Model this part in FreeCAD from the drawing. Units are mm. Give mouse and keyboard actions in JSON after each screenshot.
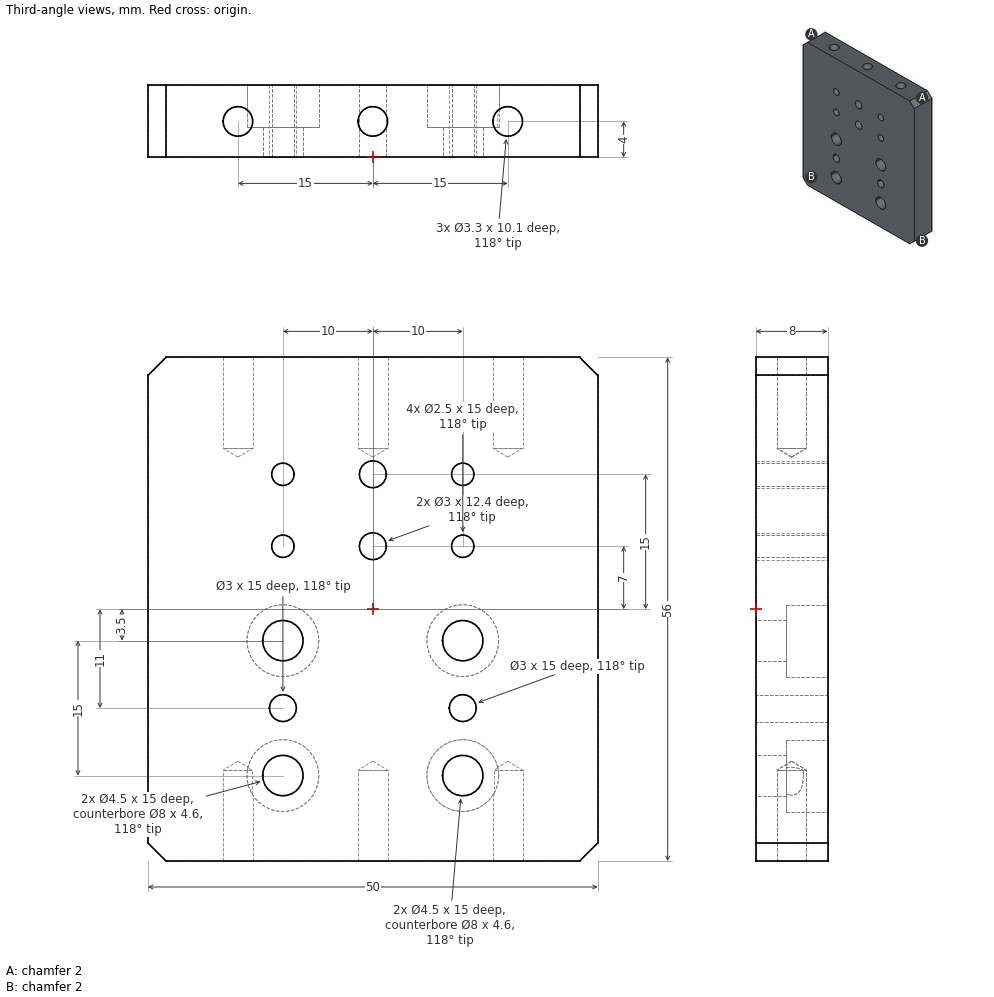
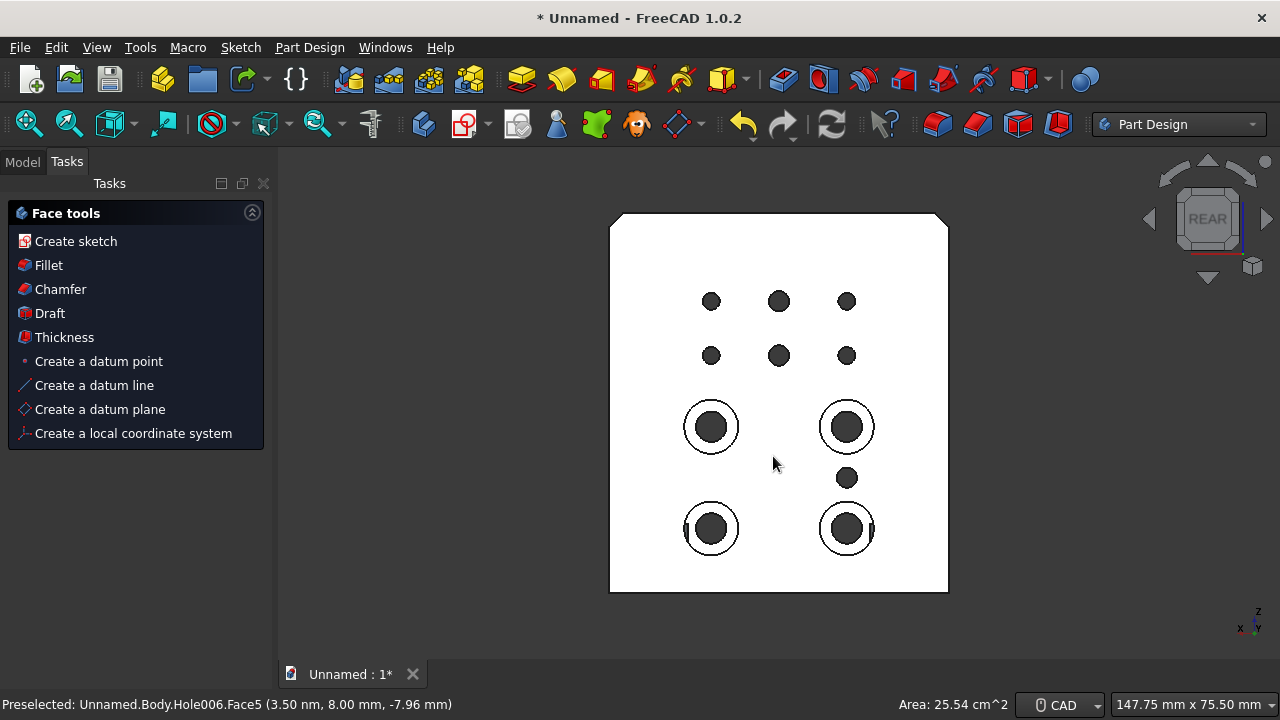
{"action": "left_click", "coordinate": [464, 124]}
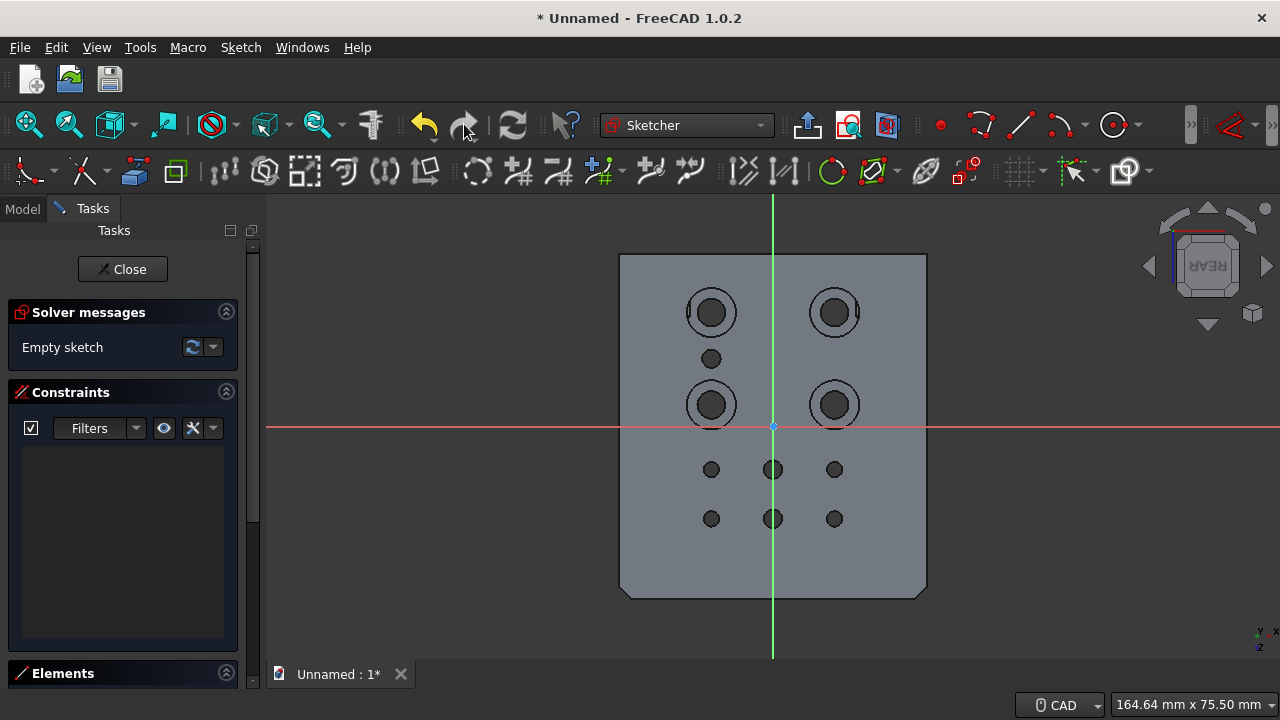
{"action": "scroll", "coordinate": [843, 354], "scroll_direction": "up", "scroll_amount": 14}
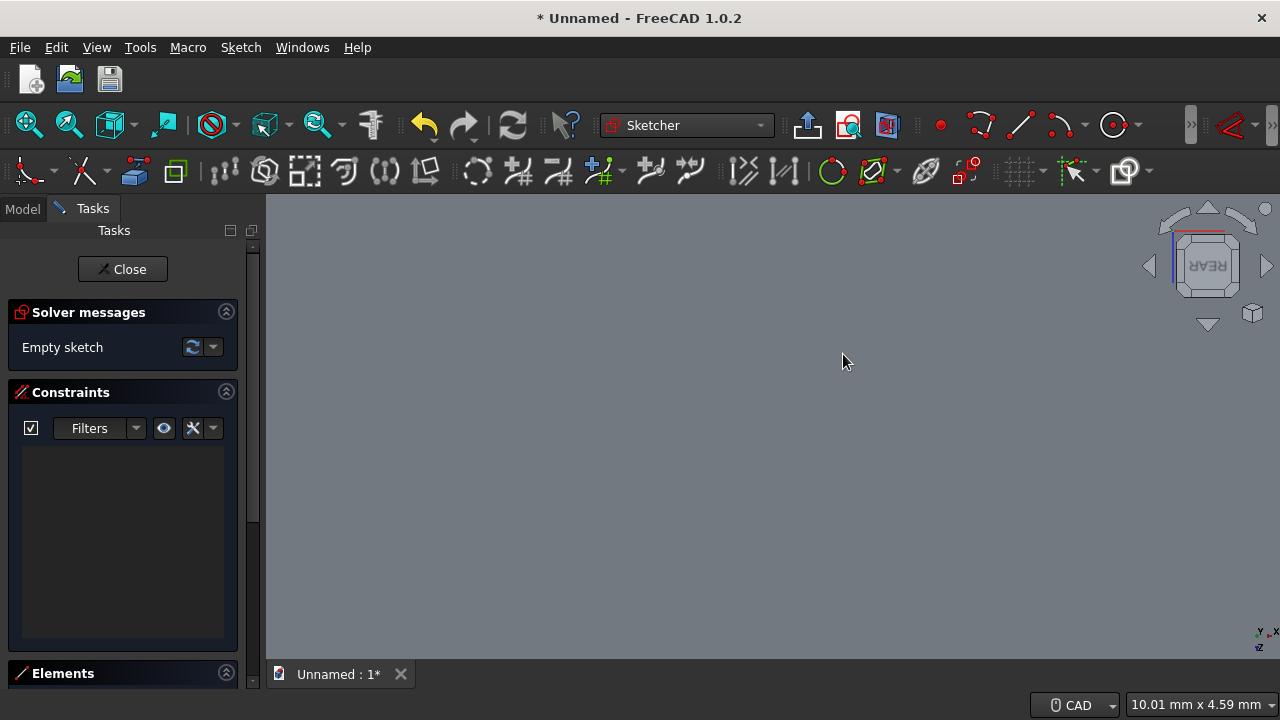
{"action": "left_click", "coordinate": [1114, 126]}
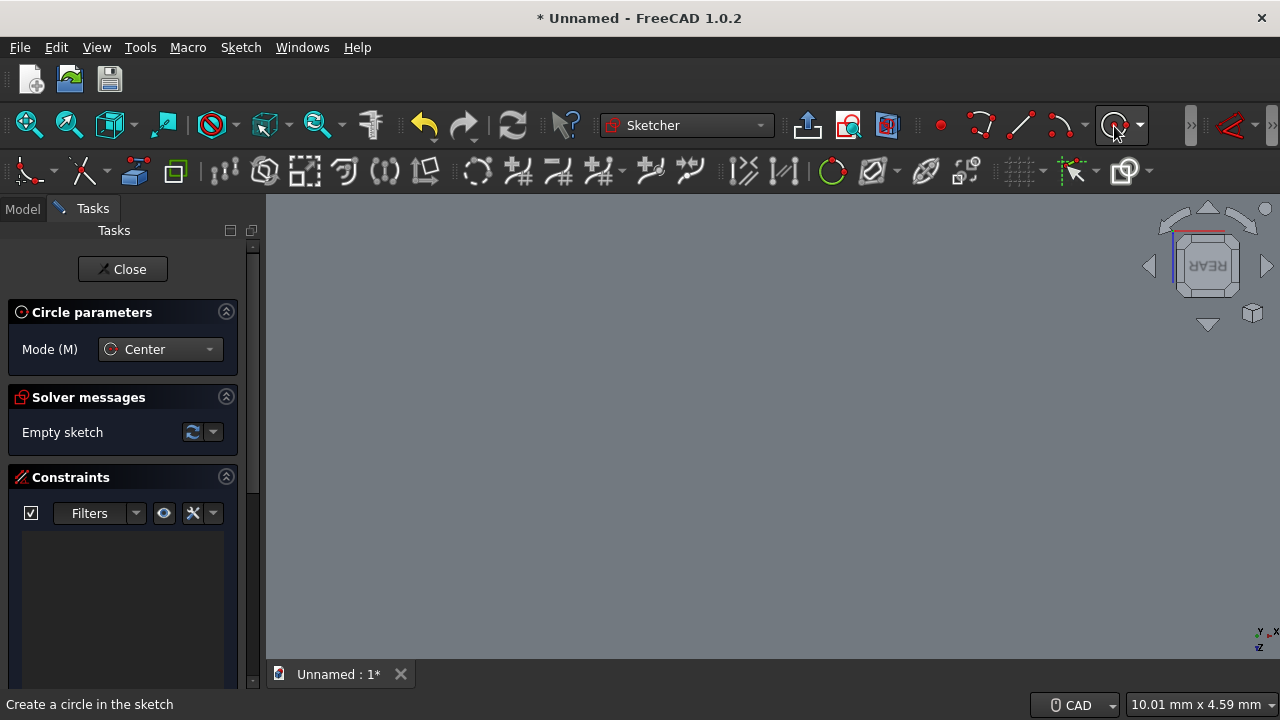
{"action": "left_click", "coordinate": [696, 427]}
{"action": "mouse_move", "coordinate": [803, 319]}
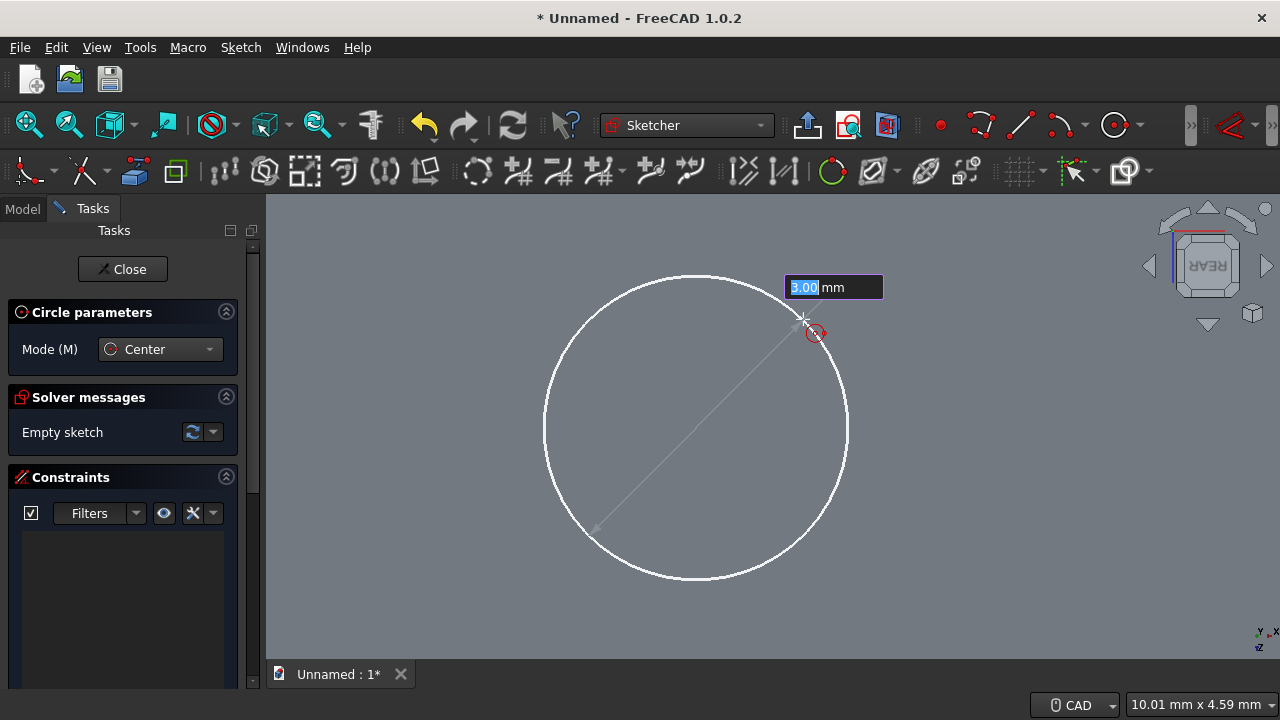
{"action": "type", "text": "3"}
{"action": "key", "text": "Return"}
{"action": "key", "text": "Escape"}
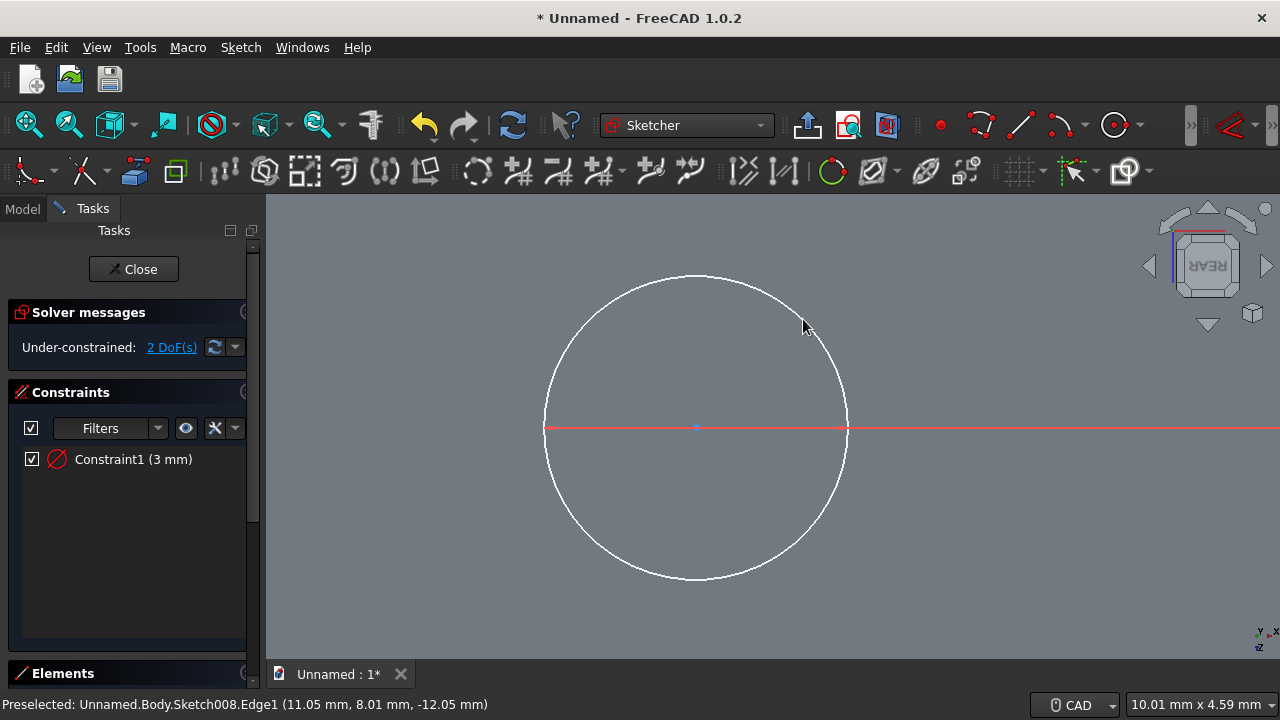
{"action": "key", "text": "d"}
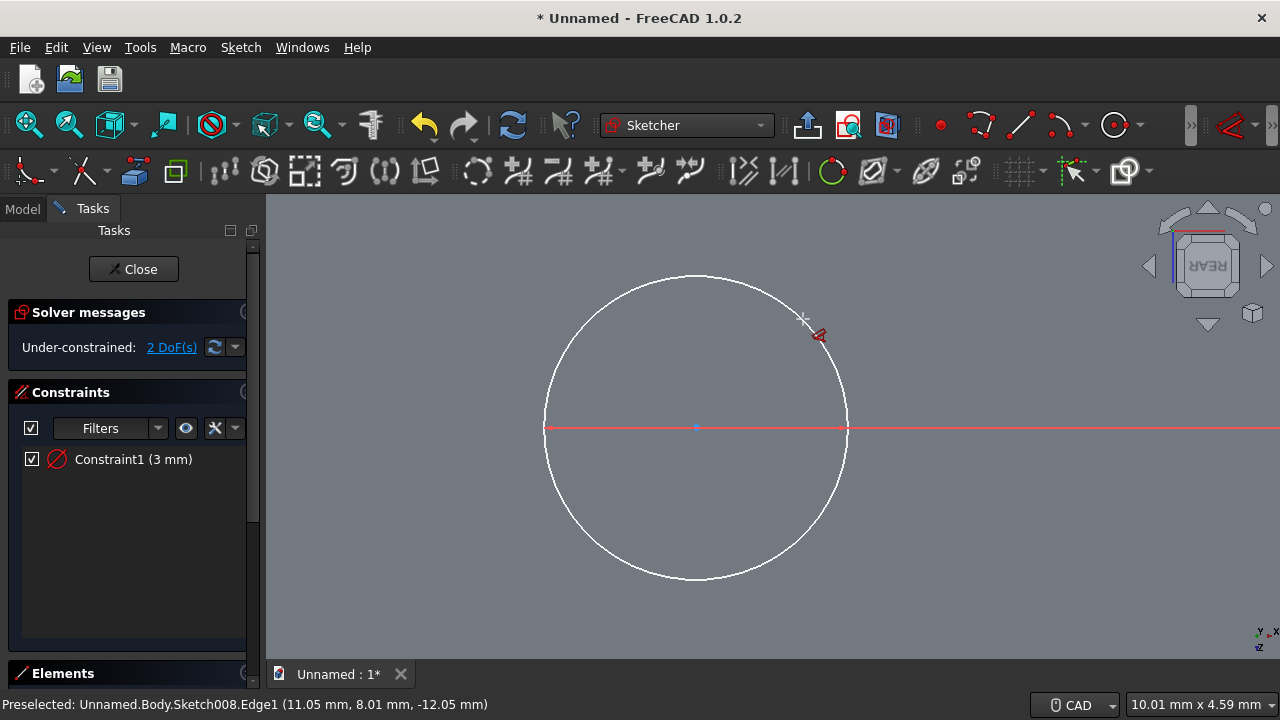
{"action": "left_click", "coordinate": [696, 428]}
{"action": "left_click", "coordinate": [495, 394]}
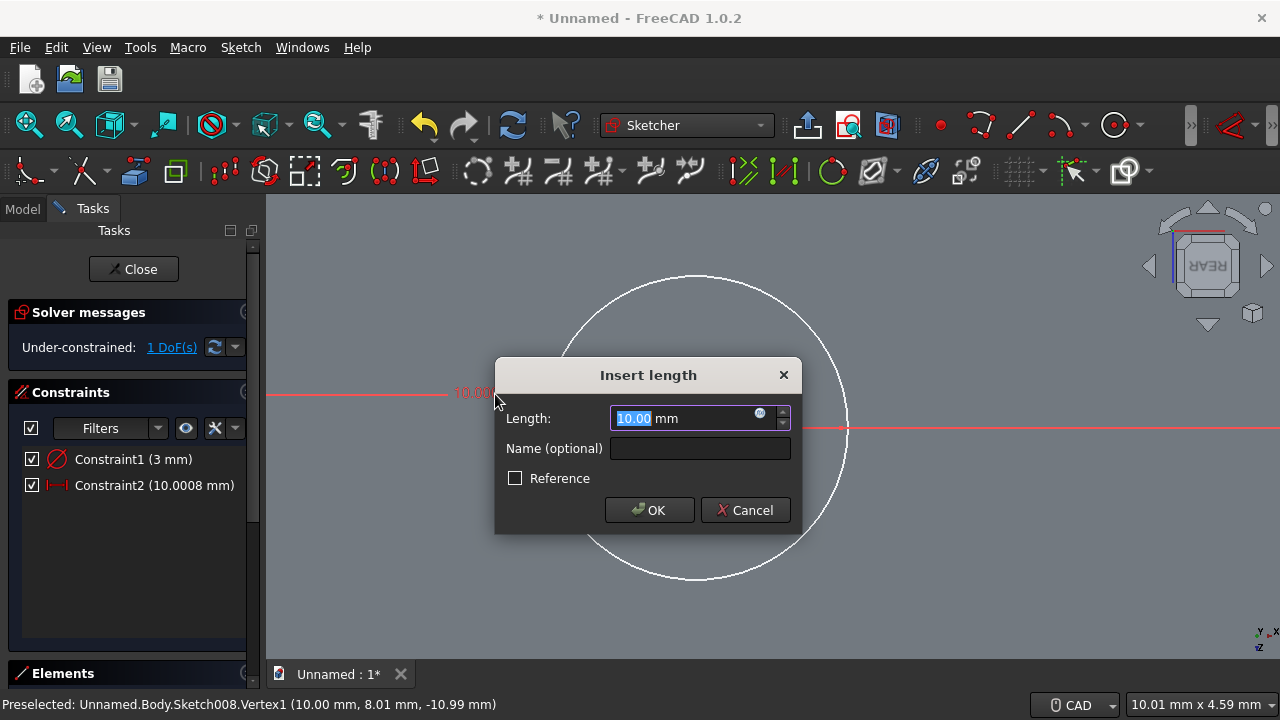
{"action": "type", "text": "10"}
{"action": "key", "text": "Return"}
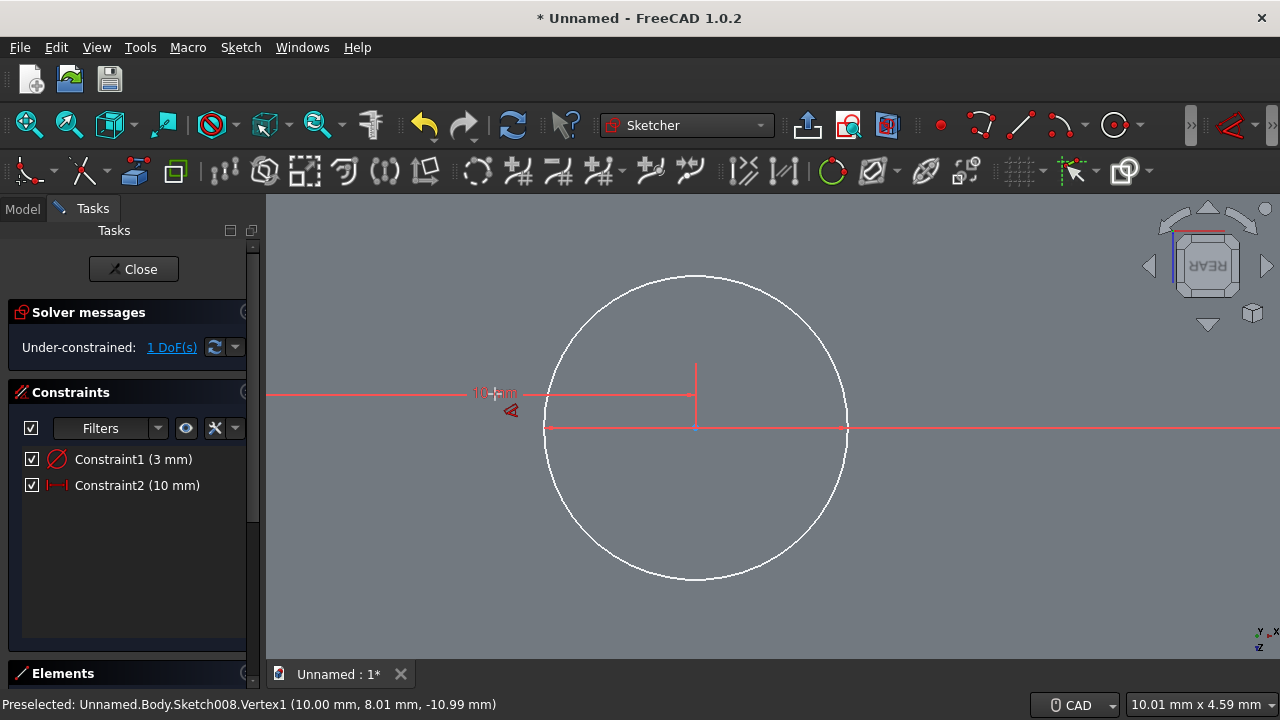
{"action": "left_click", "coordinate": [696, 428]}
{"action": "left_click", "coordinate": [730, 529]}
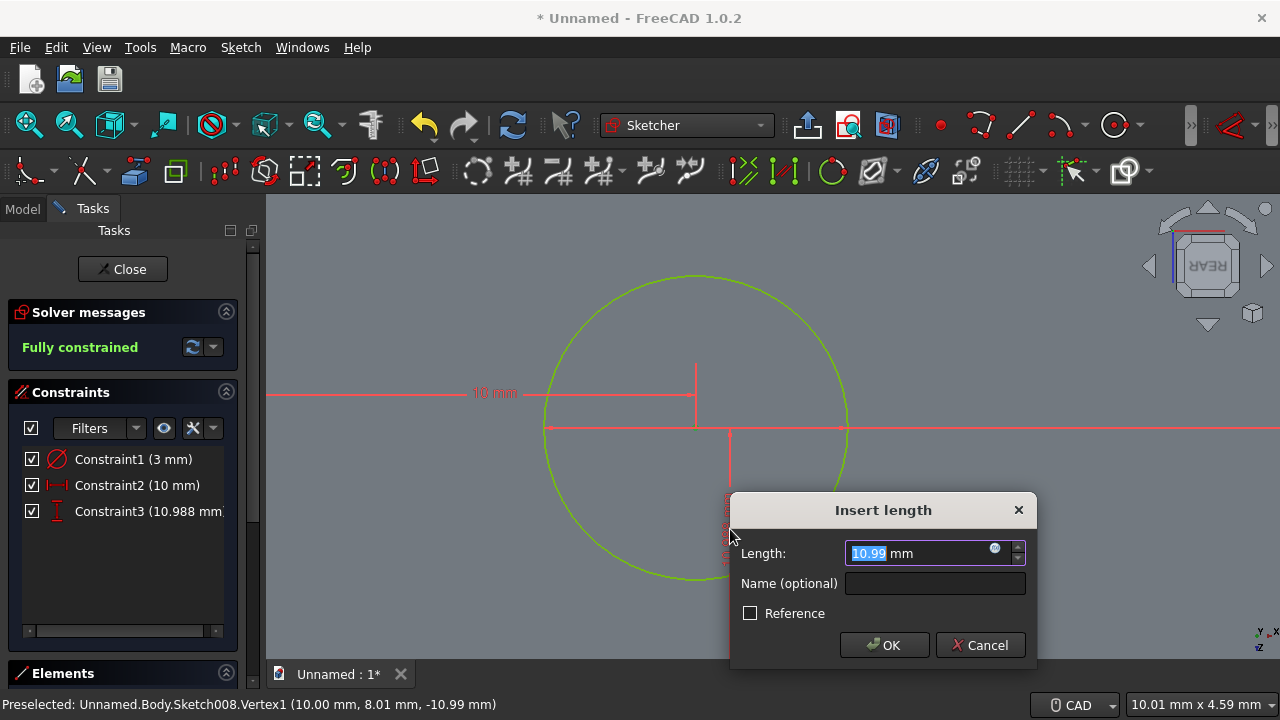
{"action": "type", "text": "11"}
{"action": "key", "text": "Return"}
{"action": "key", "text": "Escape"}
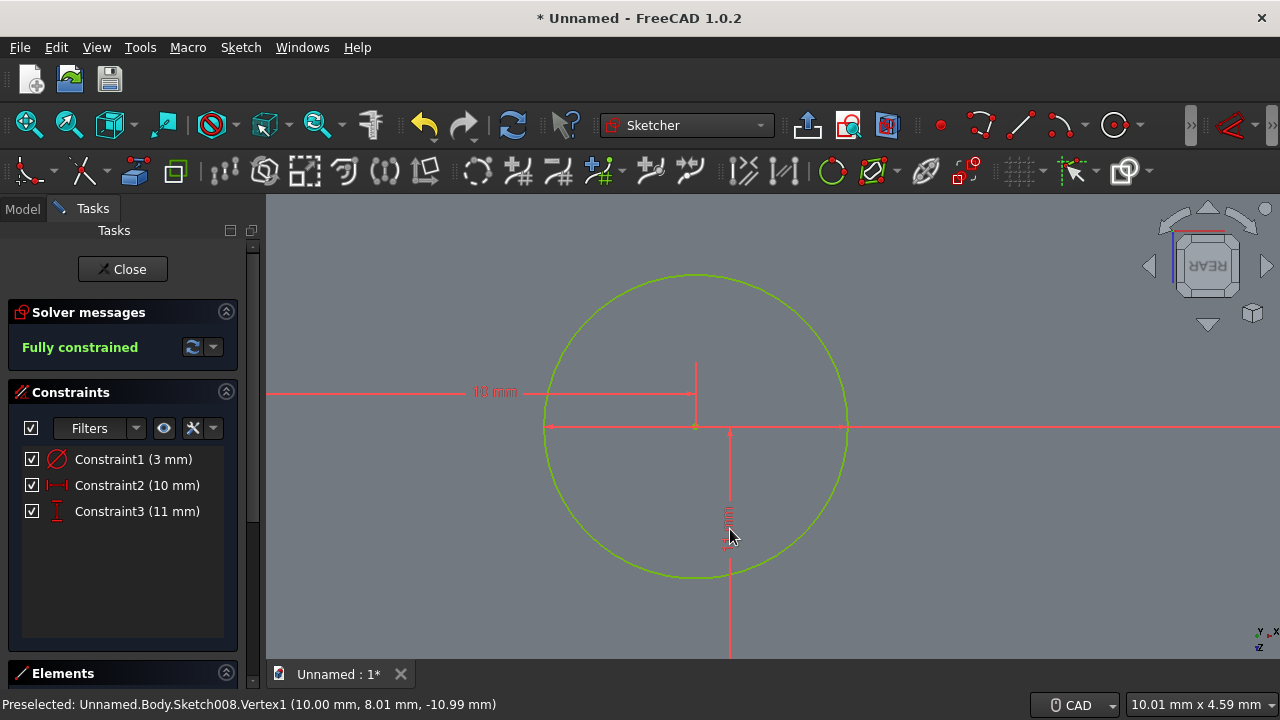
{"action": "left_click", "coordinate": [123, 269]}